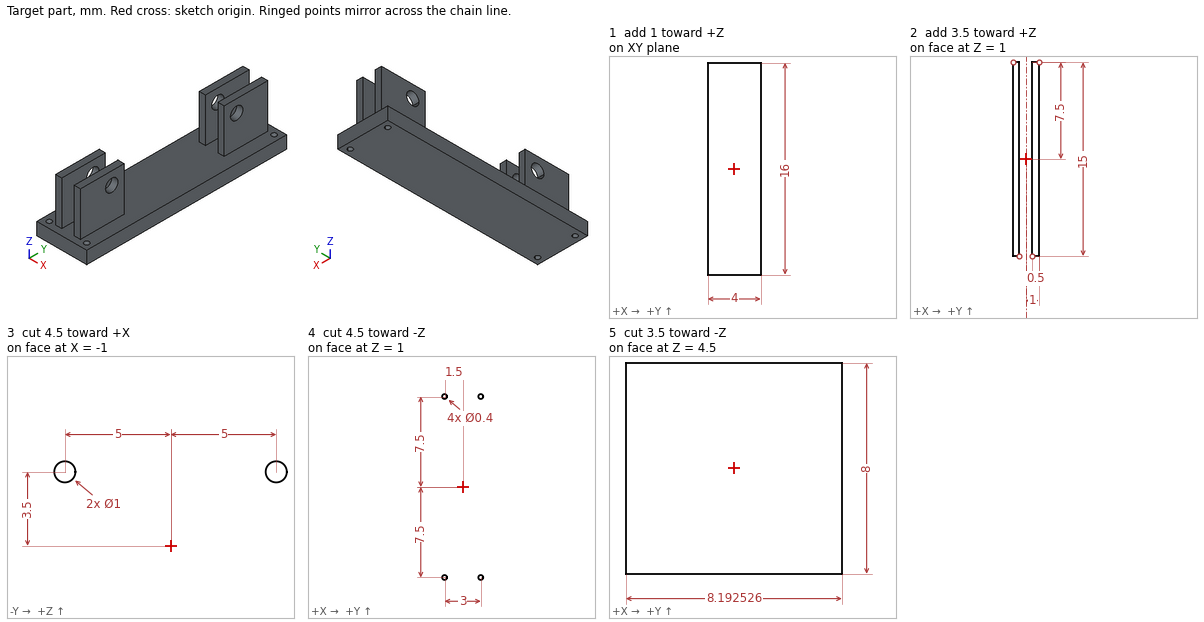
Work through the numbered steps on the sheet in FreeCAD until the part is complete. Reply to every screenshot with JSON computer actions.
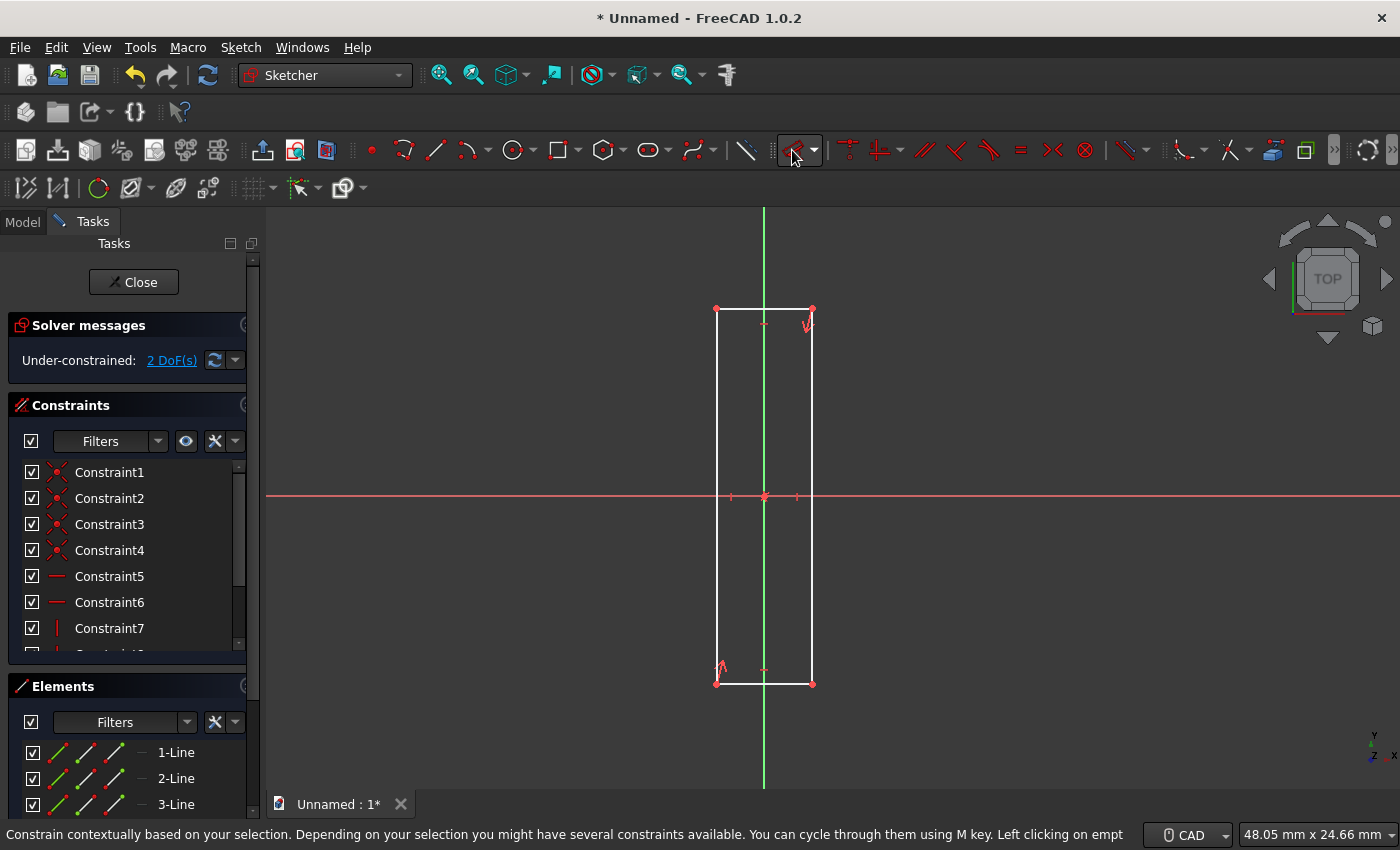
{"action": "left_click", "coordinate": [745, 684]}
{"action": "left_click", "coordinate": [743, 718]}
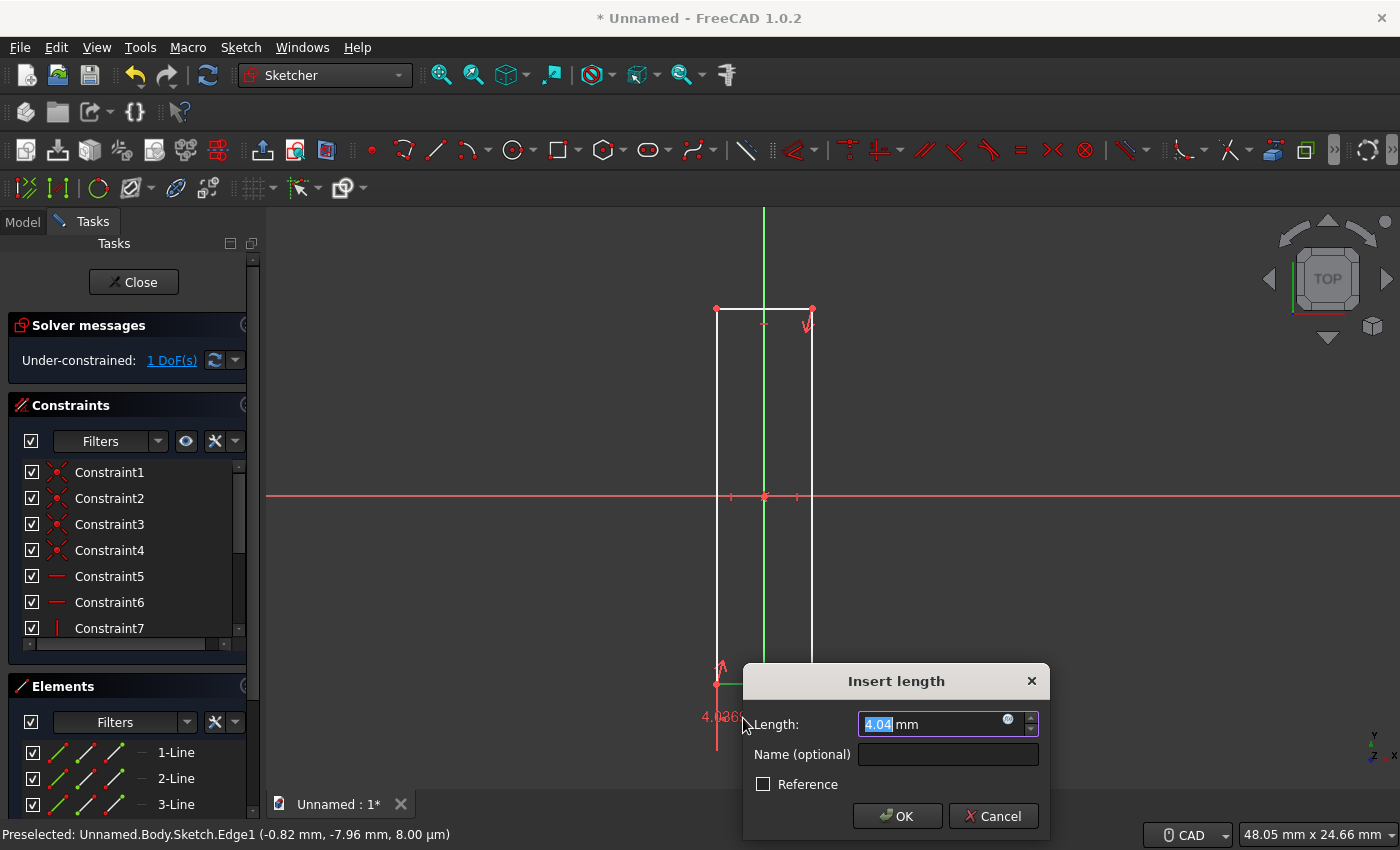
{"action": "type", "text": "4"}
{"action": "key", "text": "Return"}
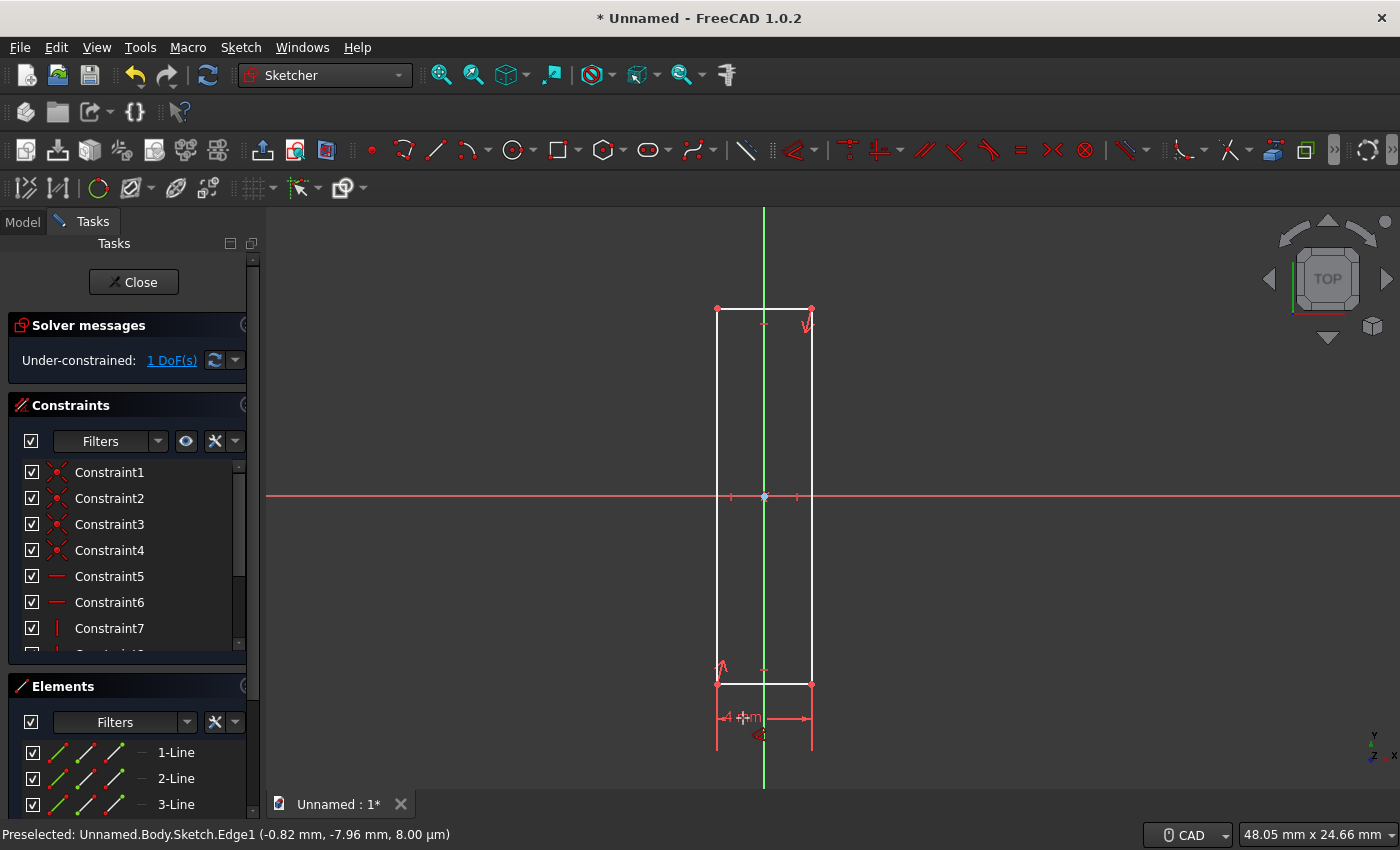
{"action": "left_click", "coordinate": [812, 572]}
{"action": "left_click", "coordinate": [846, 410]}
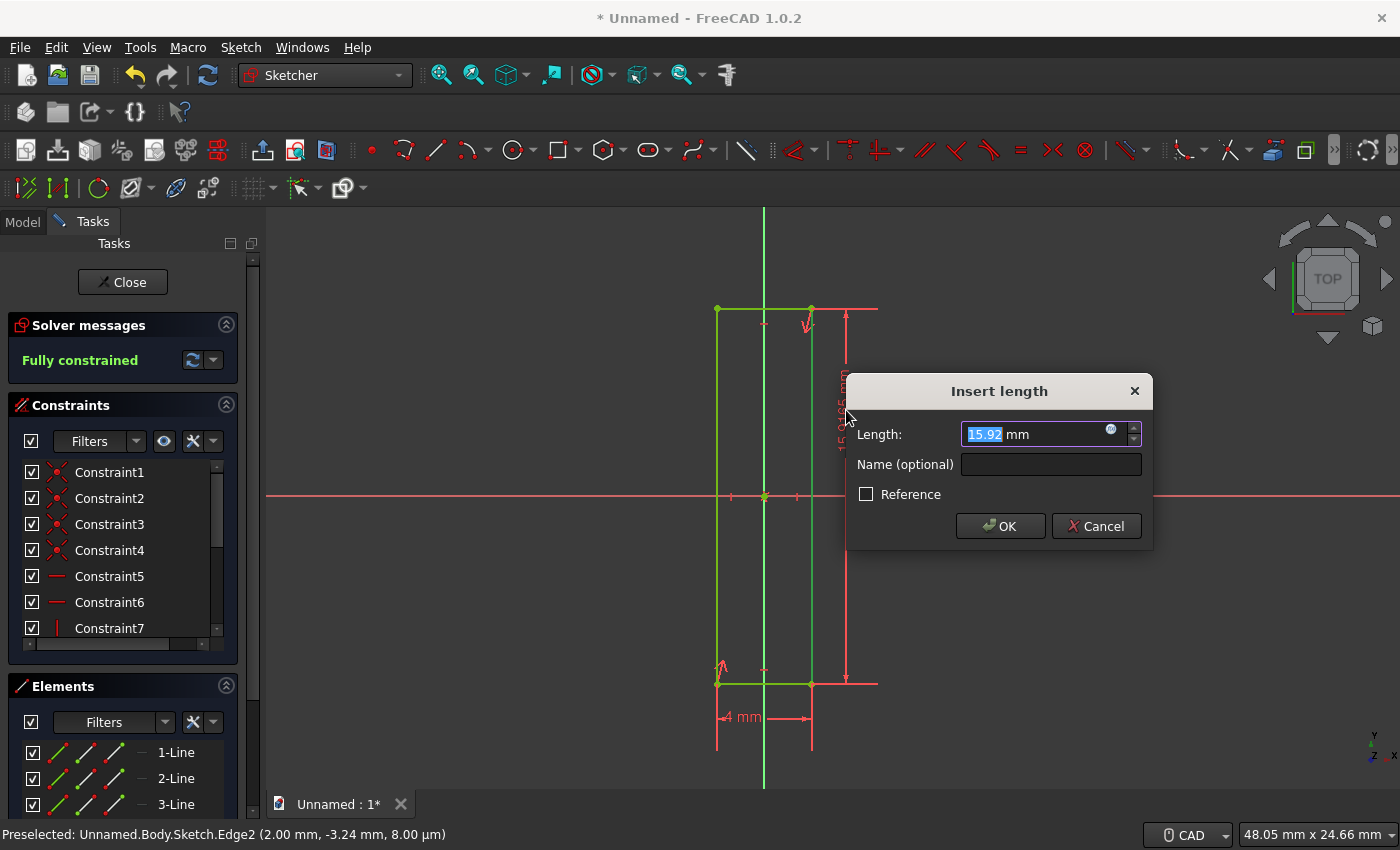
{"action": "type", "text": "16"}
{"action": "key", "text": "Return"}
{"action": "key", "text": "Escape"}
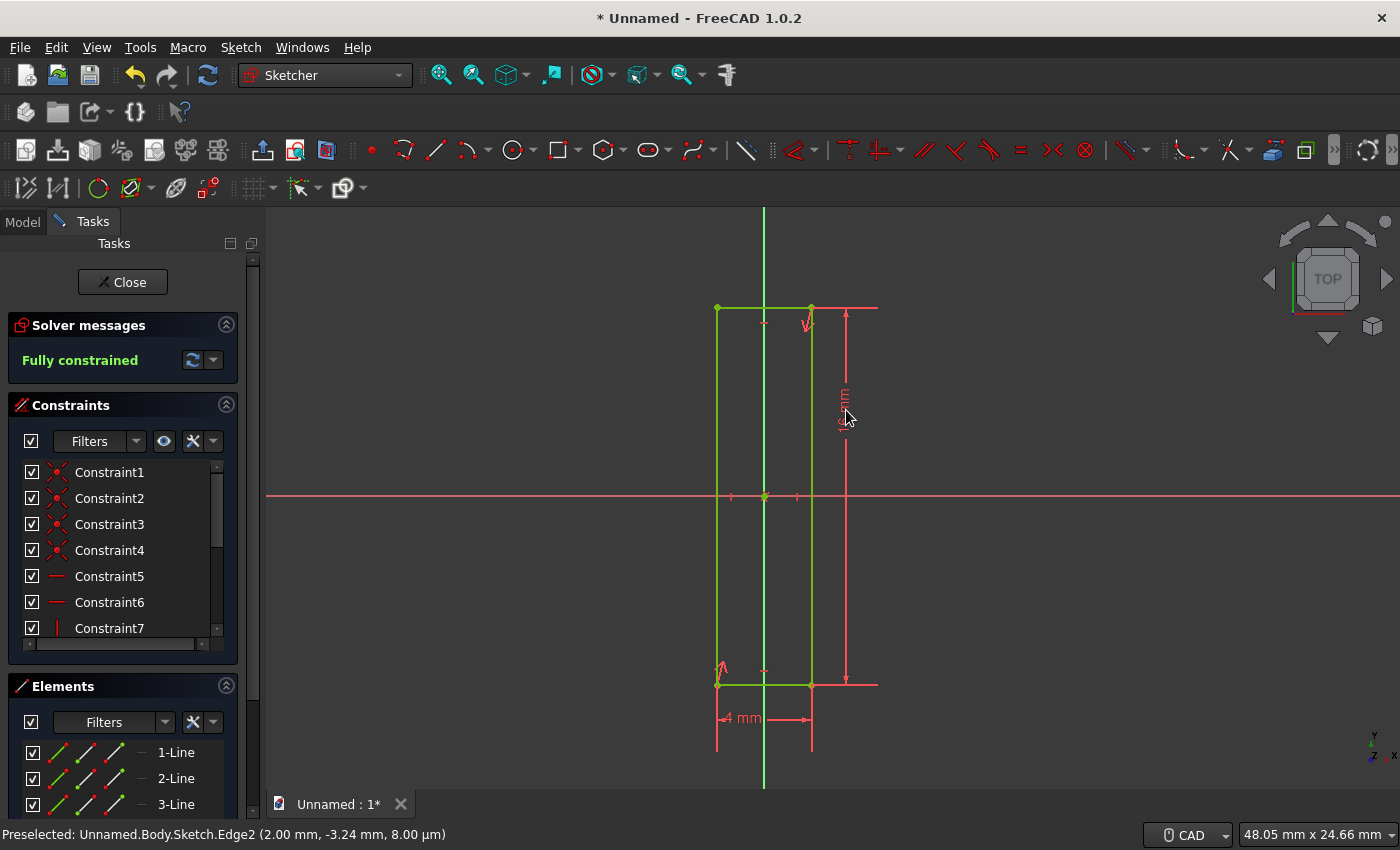
{"action": "left_click", "coordinate": [123, 282]}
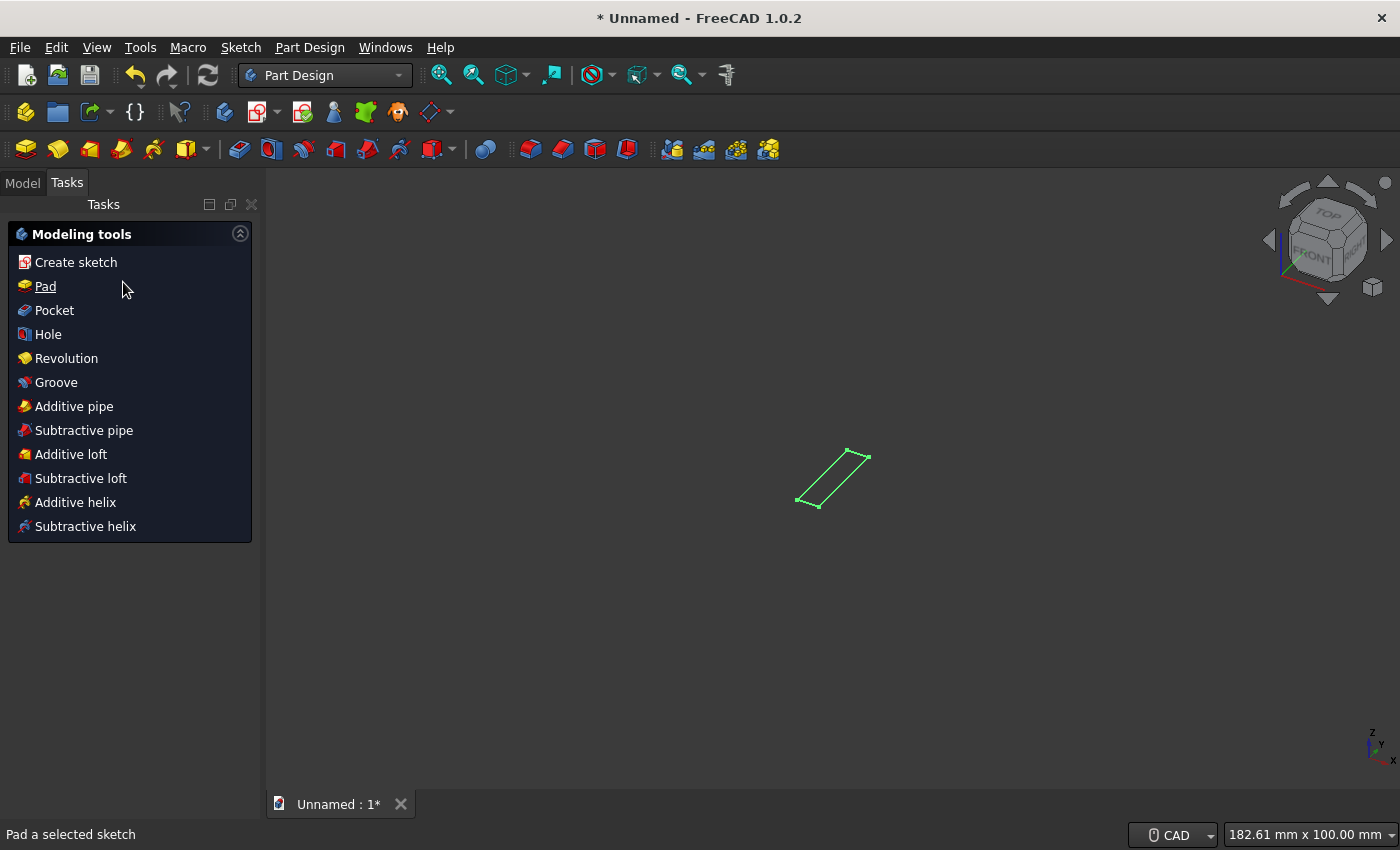
{"action": "left_click", "coordinate": [26, 150]}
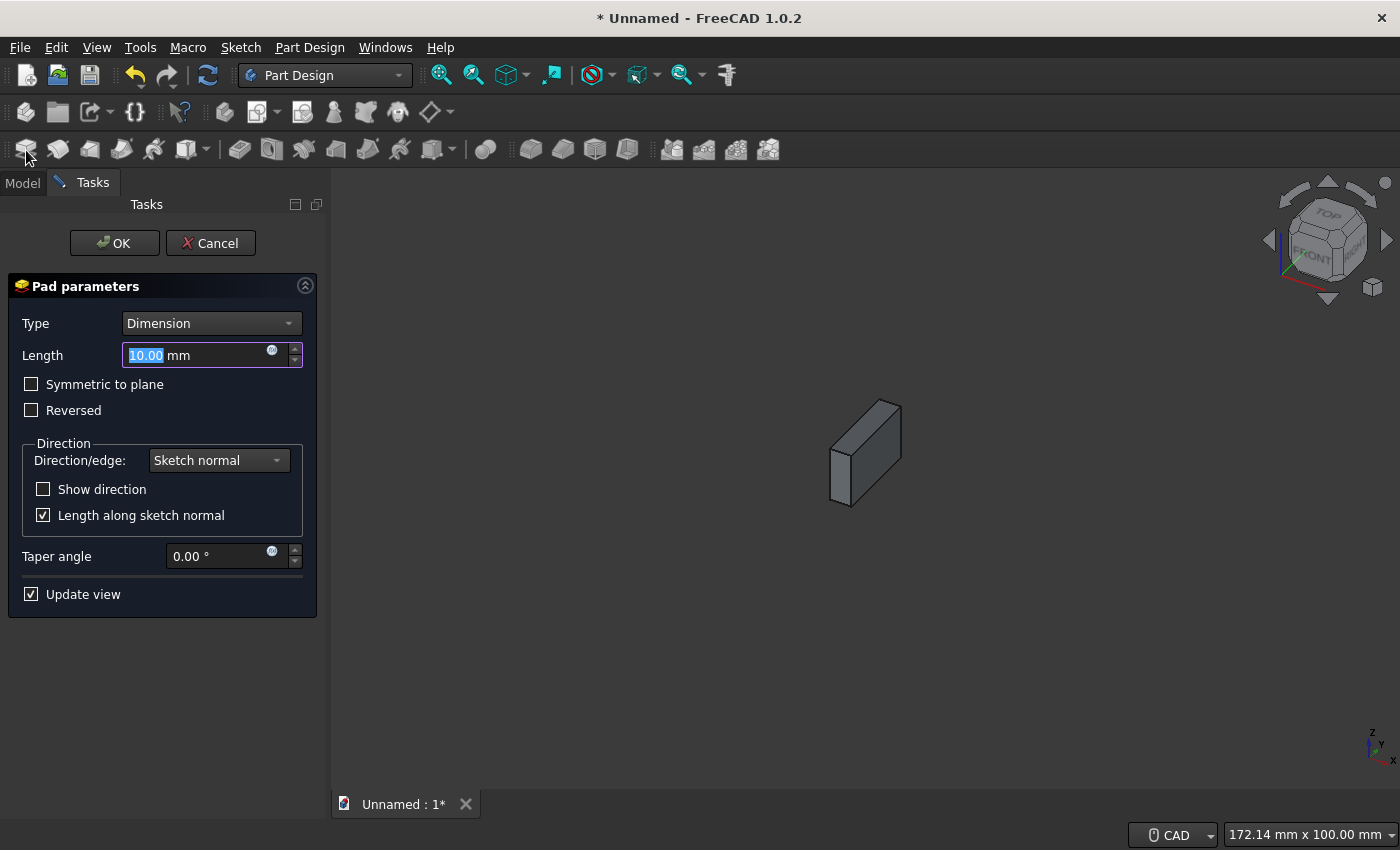
{"action": "type", "text": "1"}
{"action": "key", "text": "Tab"}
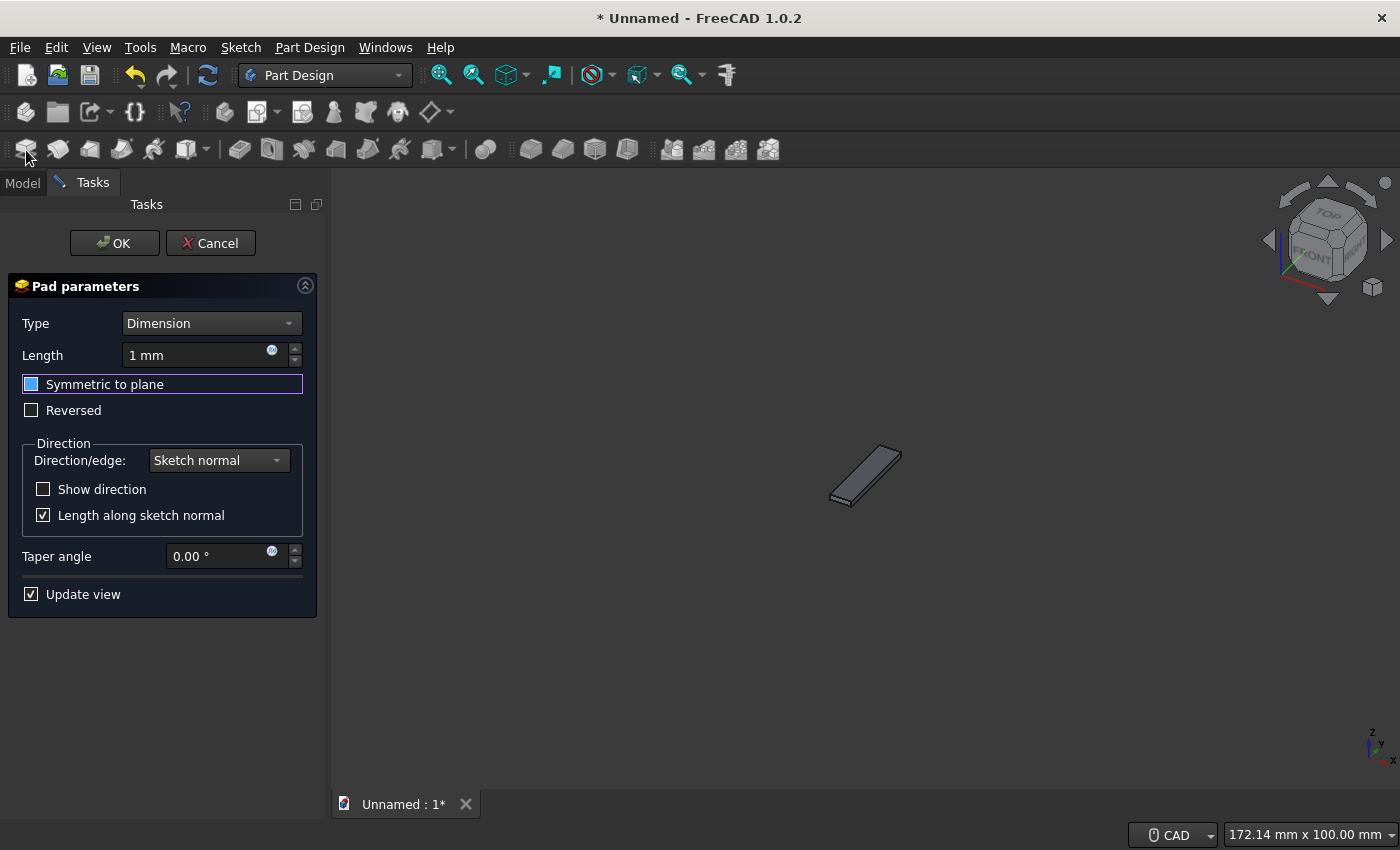
{"action": "left_click", "coordinate": [115, 243]}